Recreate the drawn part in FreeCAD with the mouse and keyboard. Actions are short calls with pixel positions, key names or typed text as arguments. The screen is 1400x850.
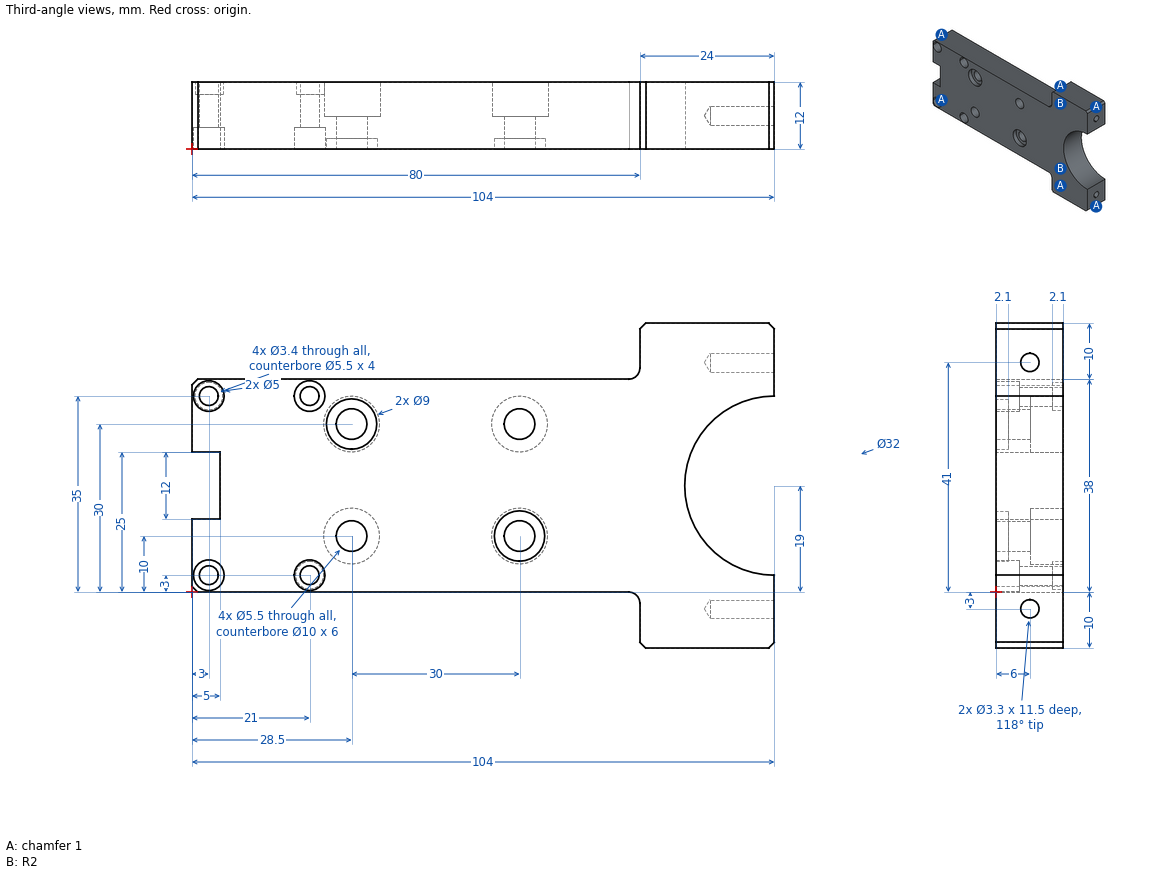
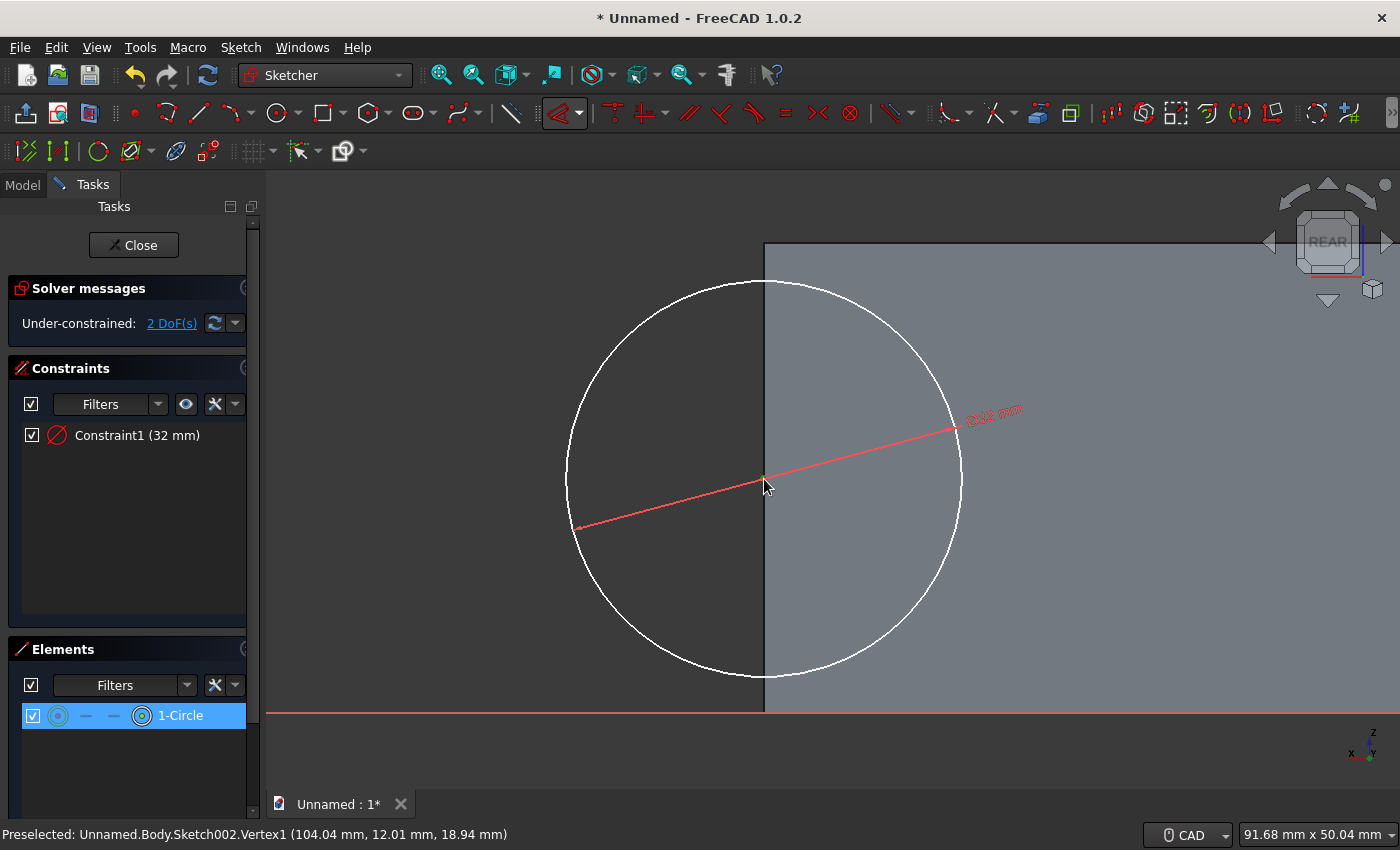
click(582, 114)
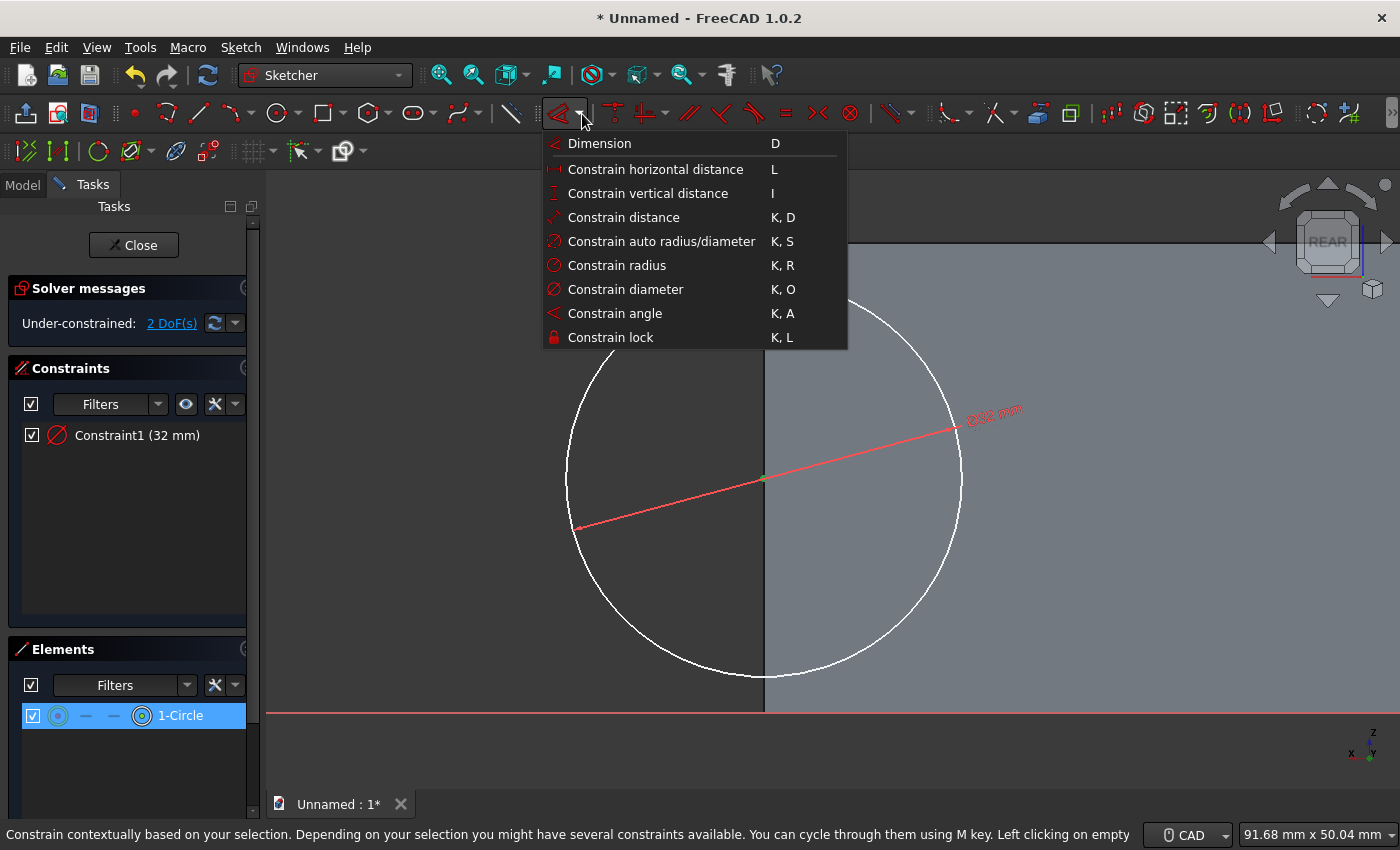
click(695, 193)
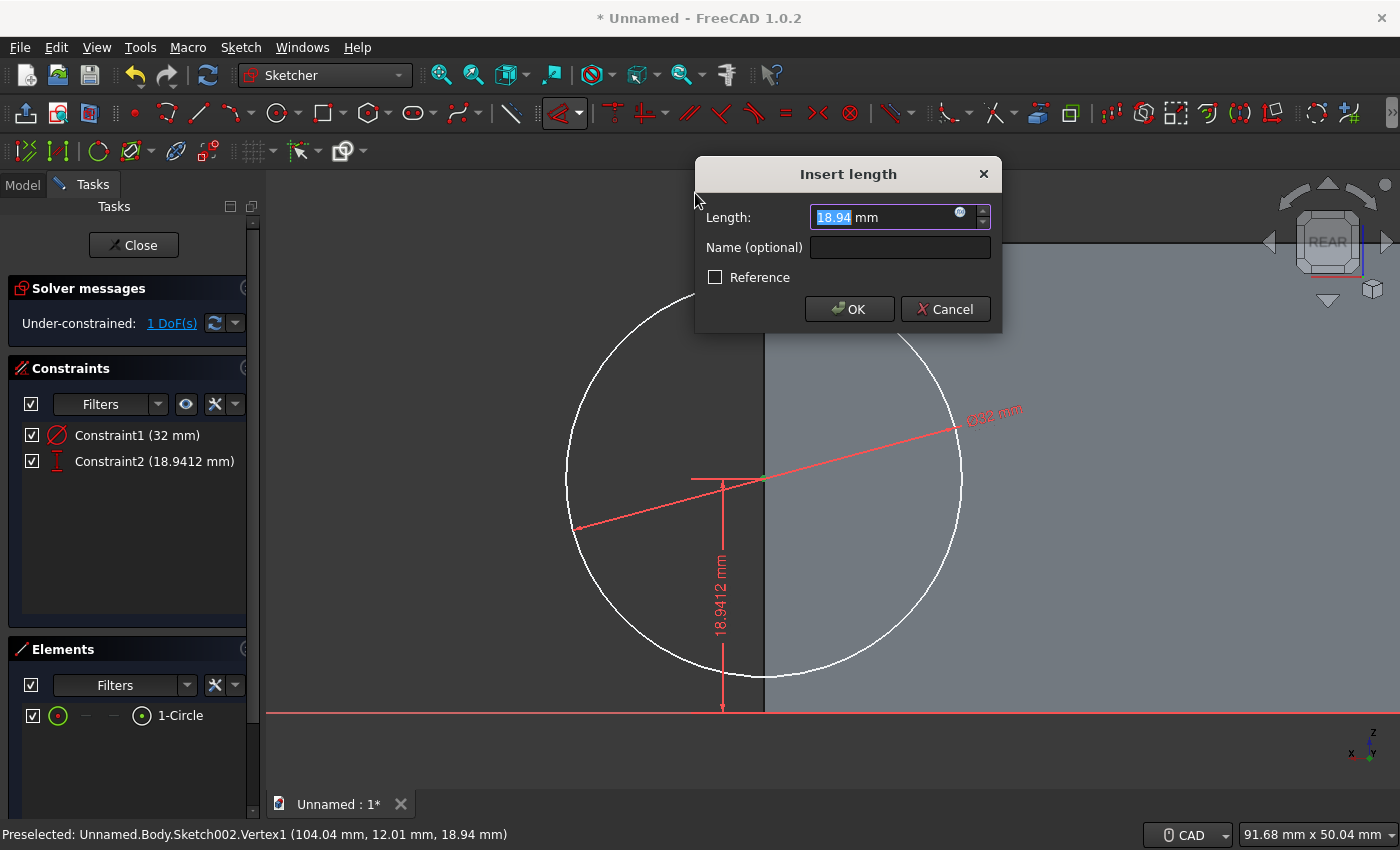
text(19)
key(Return)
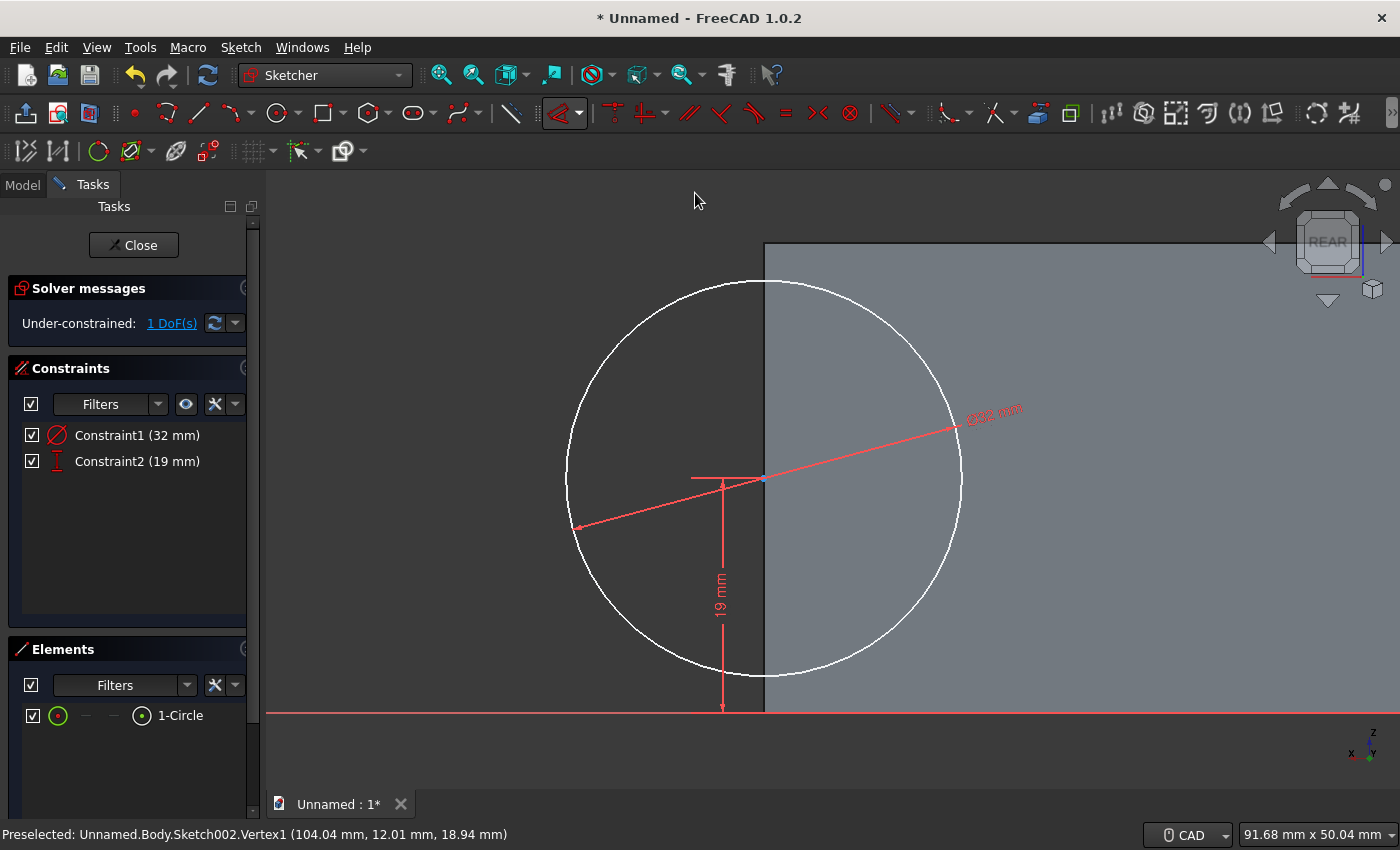
click(764, 478)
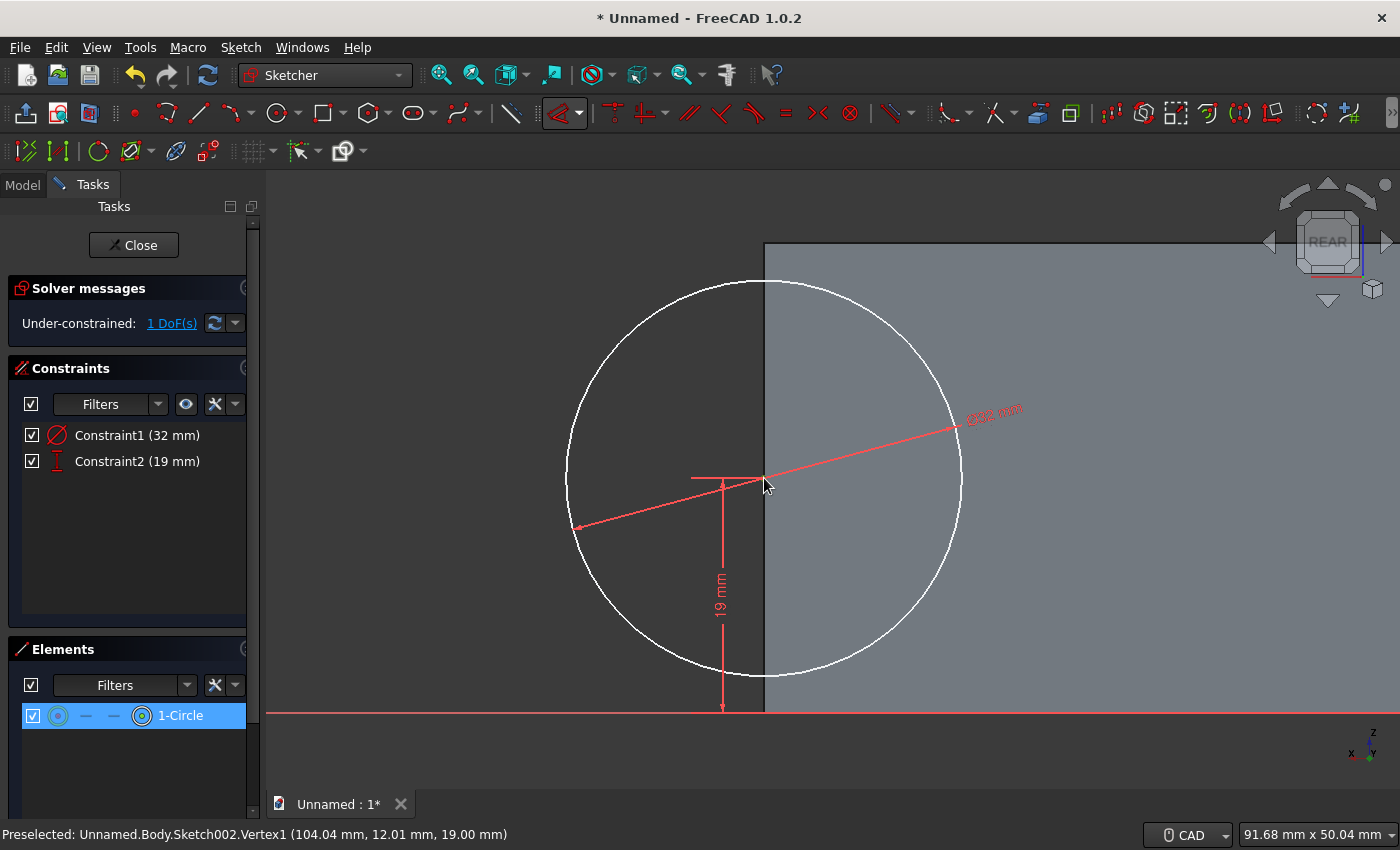
key(l)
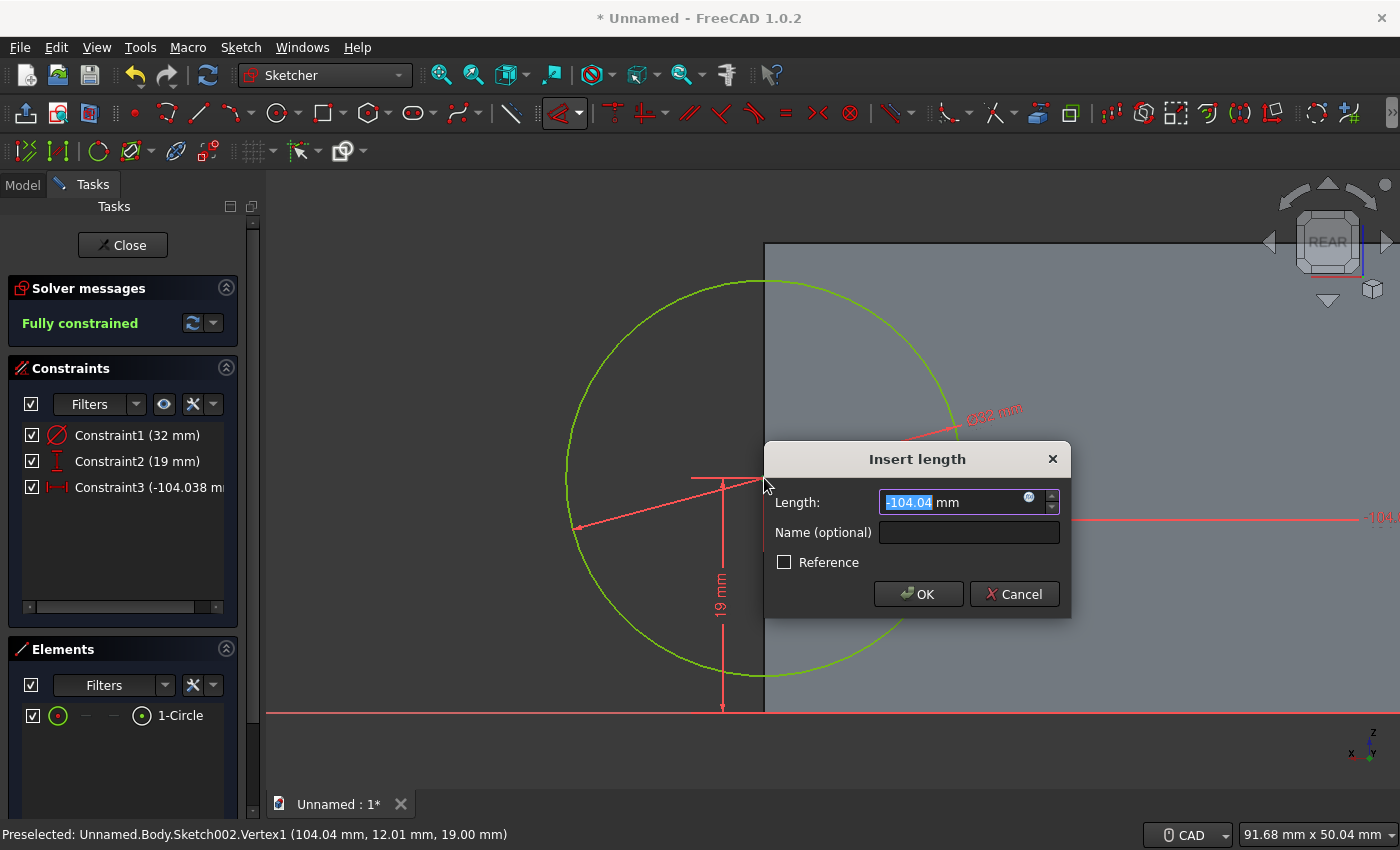
text(-104)
key(Return)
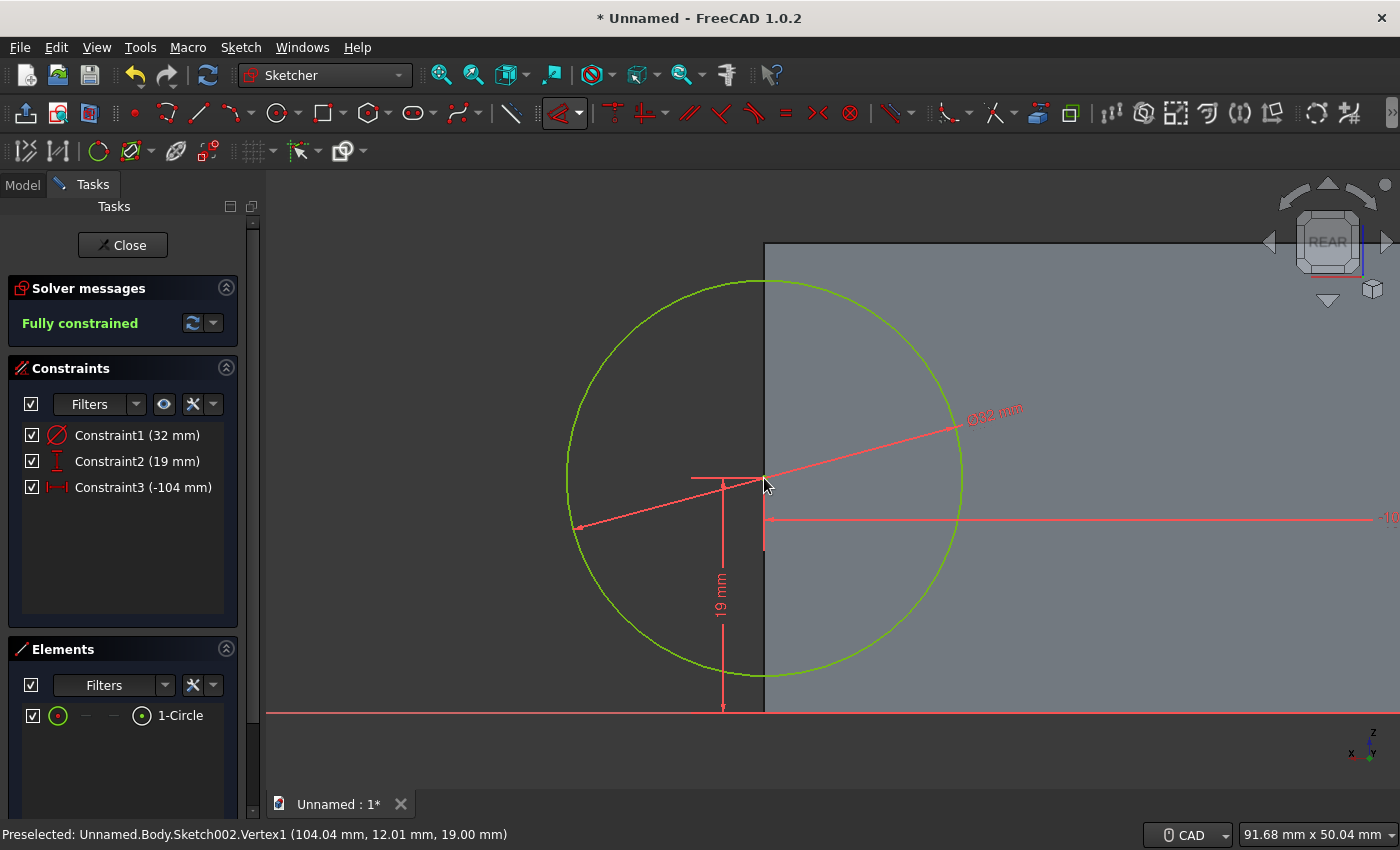
click(123, 245)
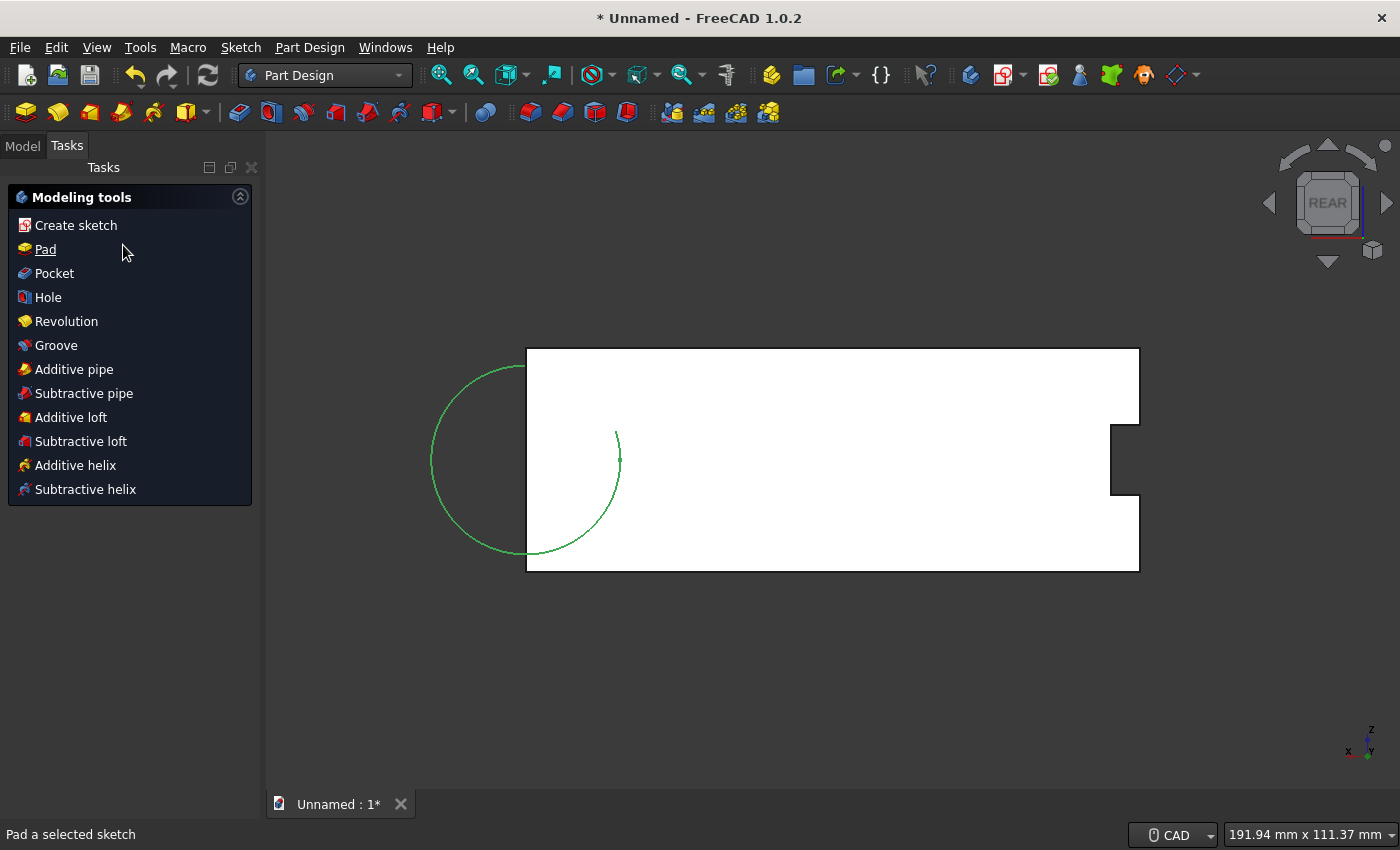
click(240, 112)